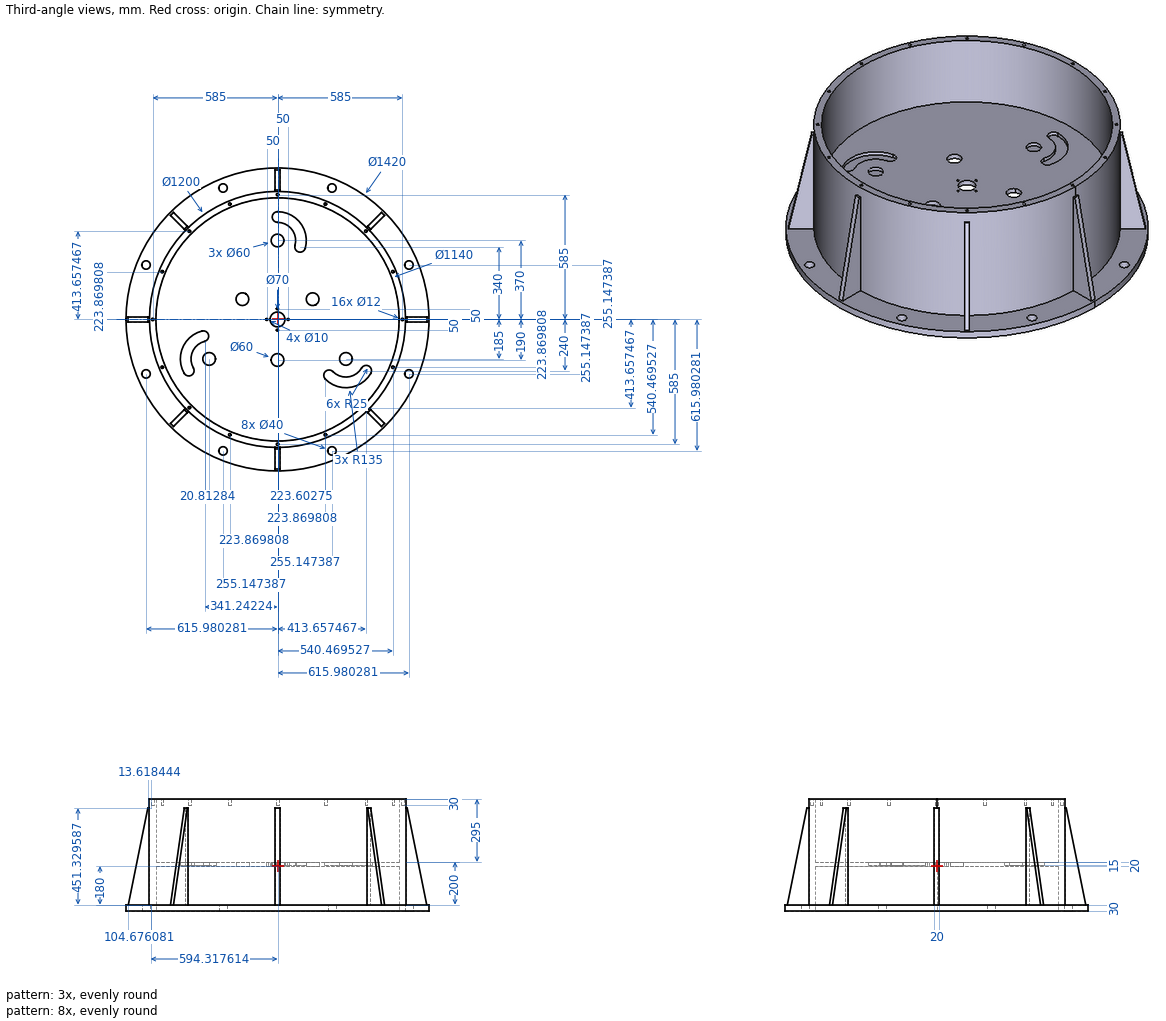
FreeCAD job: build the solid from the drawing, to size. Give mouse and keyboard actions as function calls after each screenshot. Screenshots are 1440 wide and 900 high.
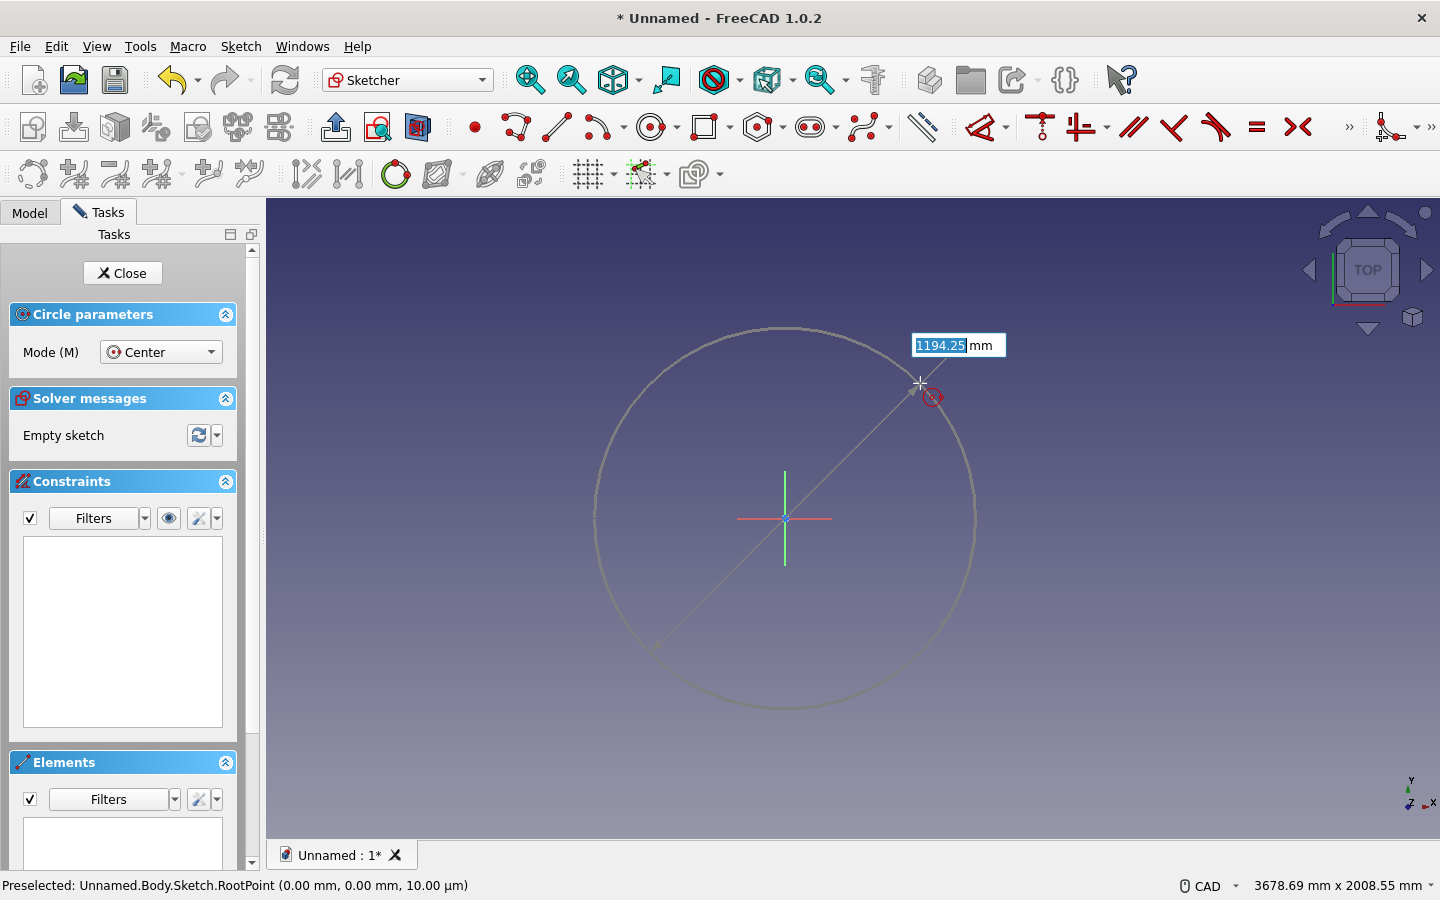
text(1200)
key(Return)
key(Escape)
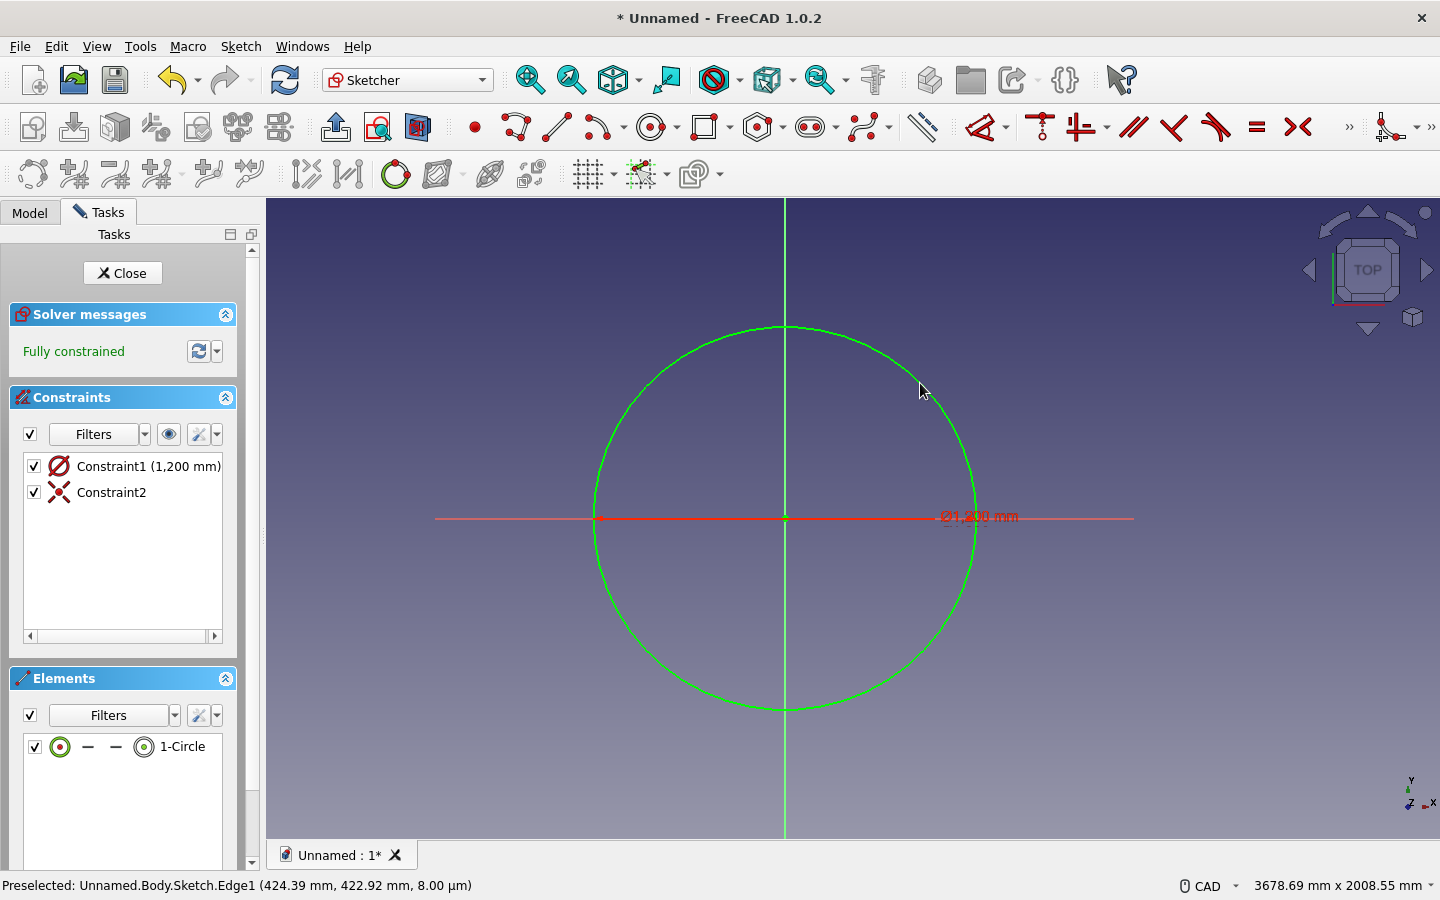
click(123, 273)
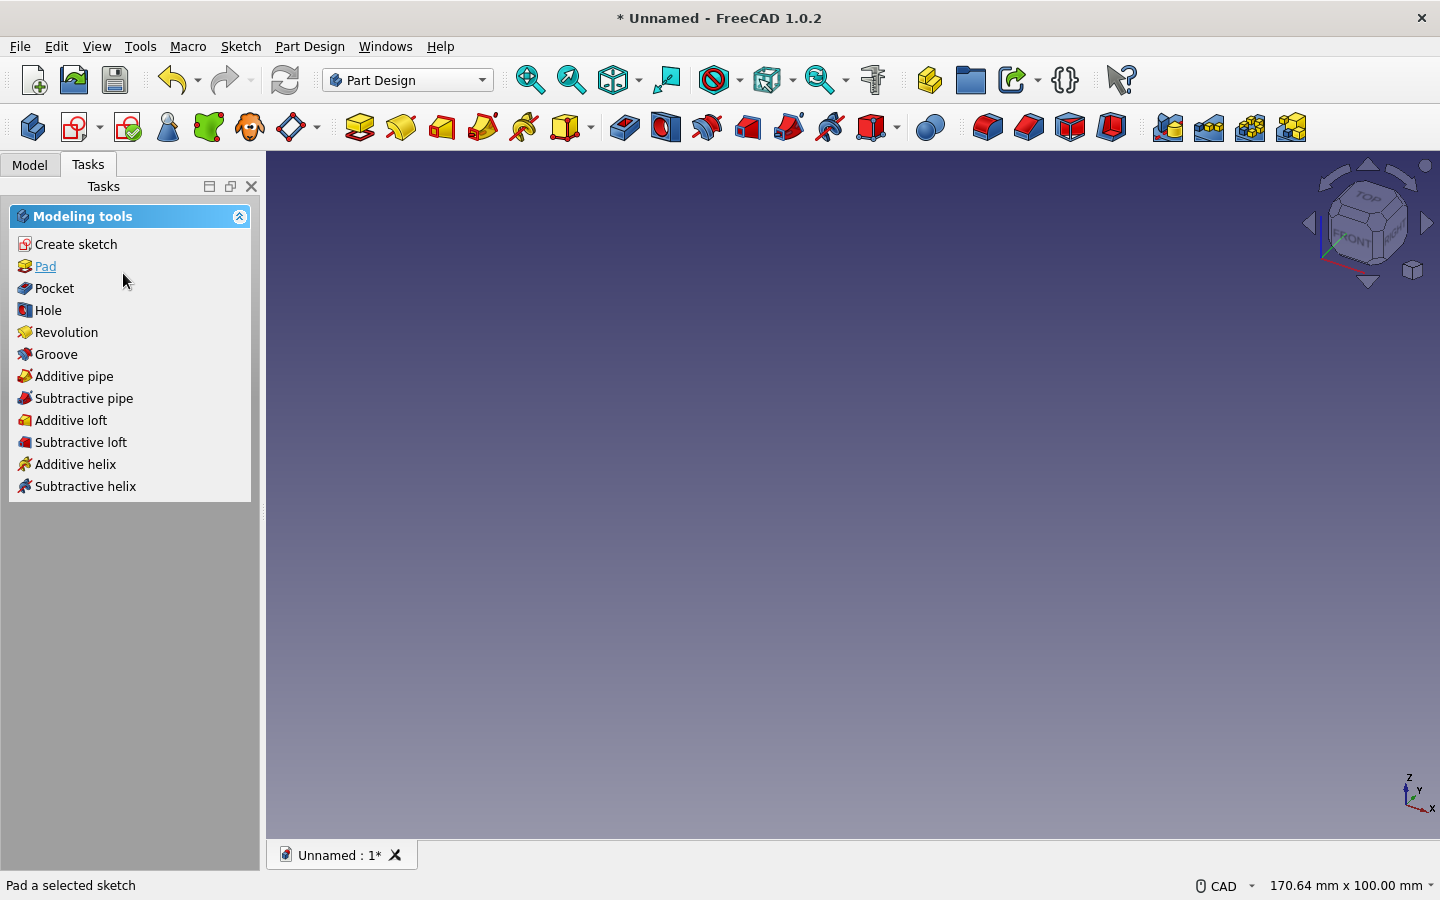
click(360, 128)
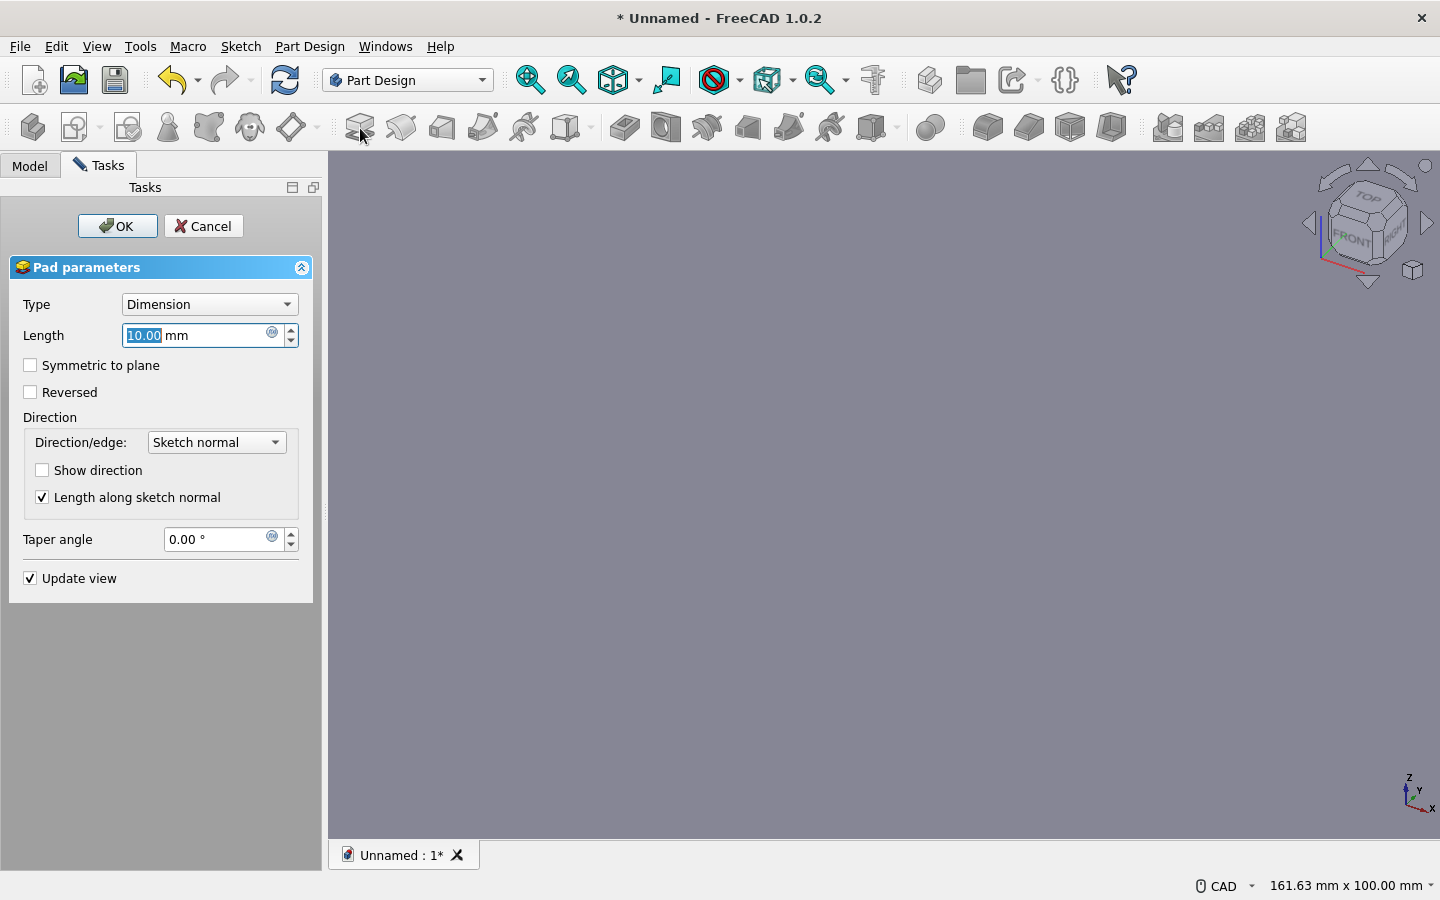
text(20)
key(Tab)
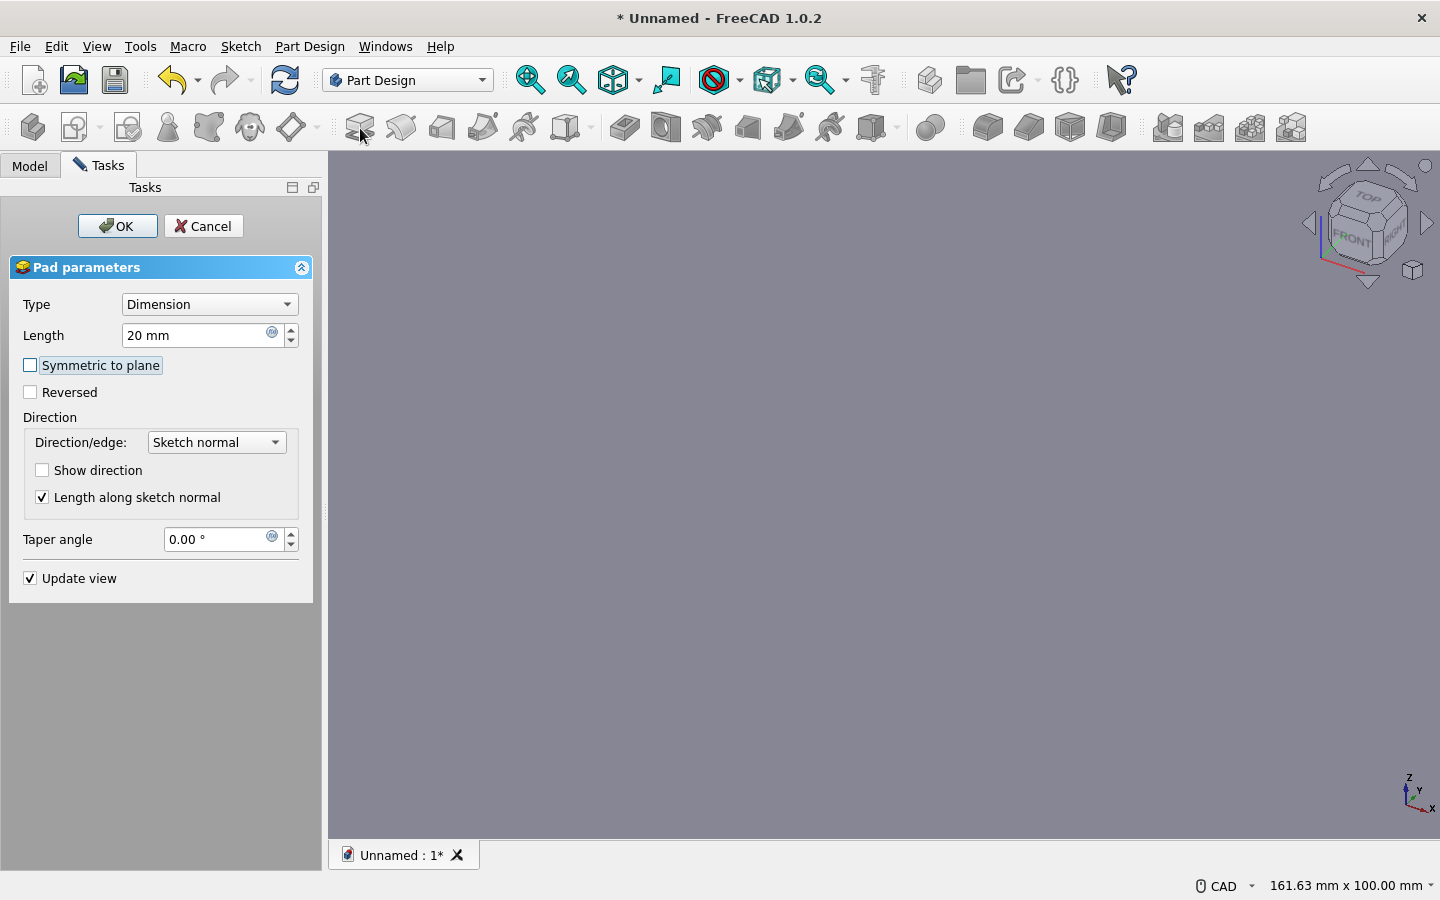
click(118, 226)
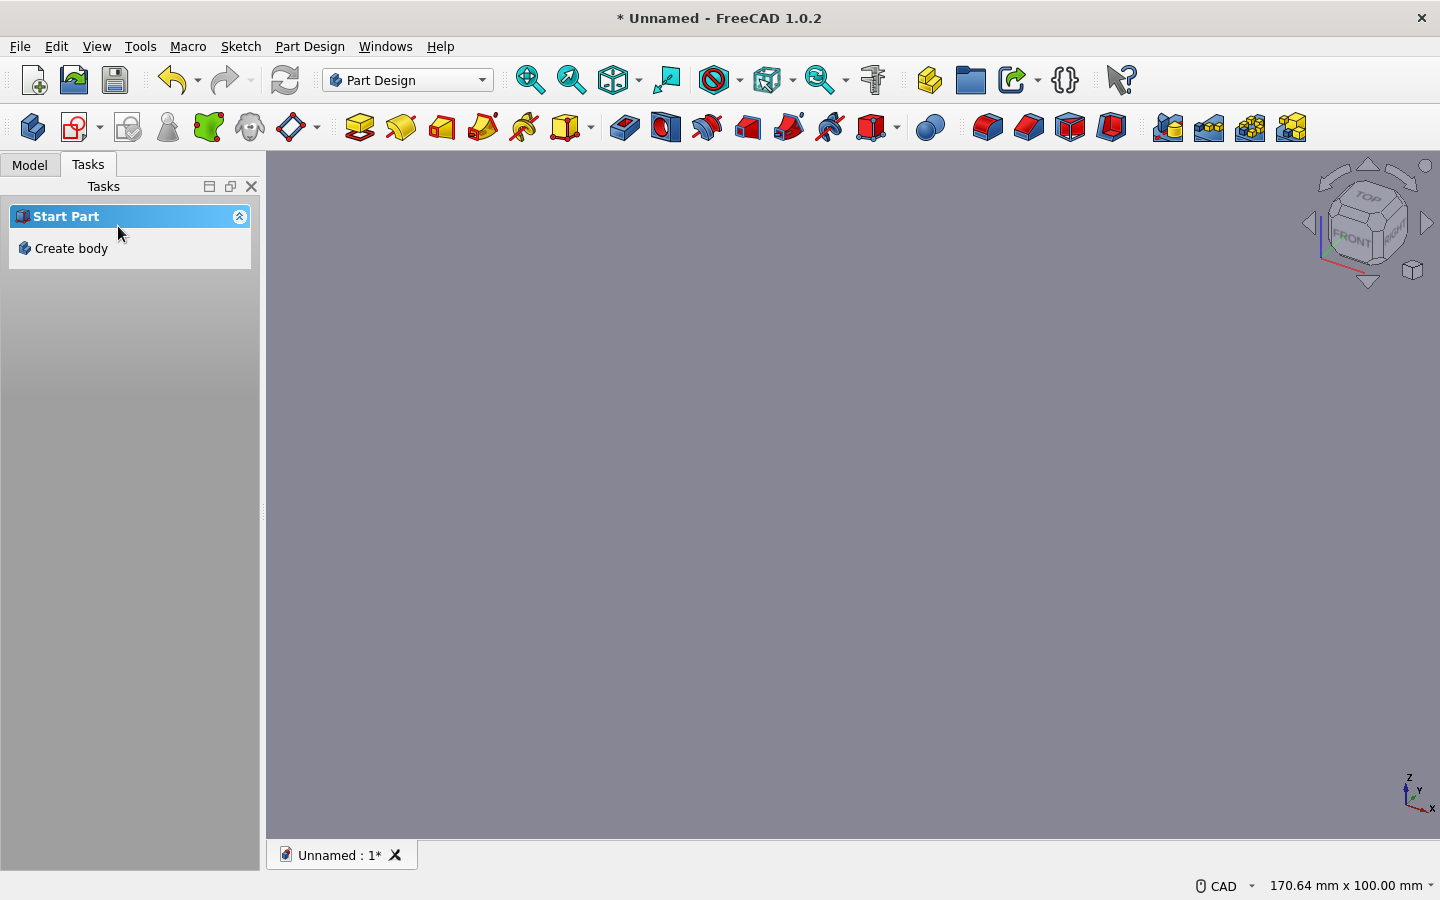
click(531, 80)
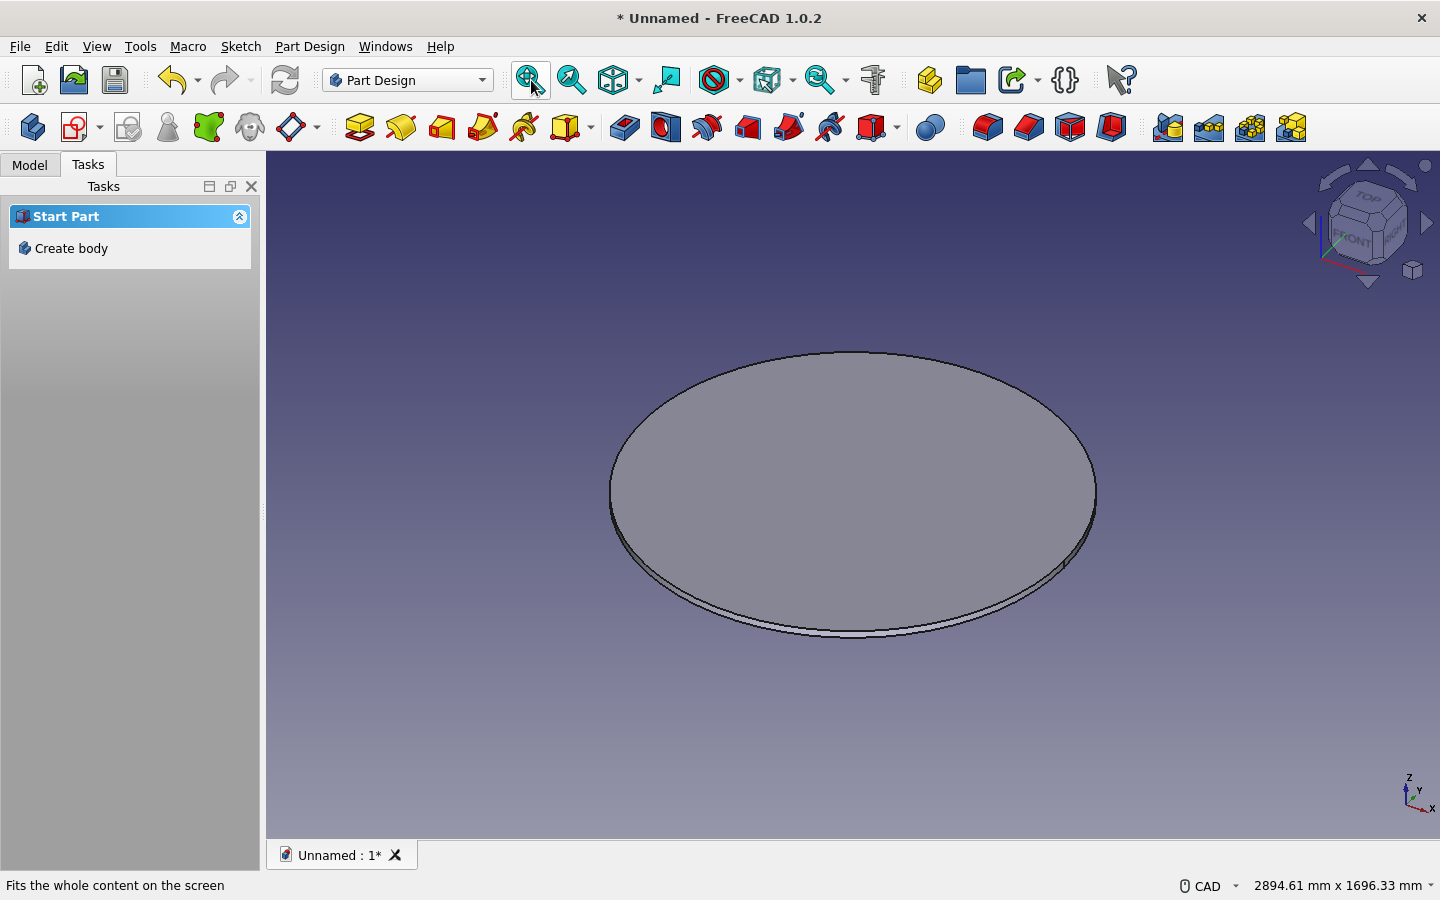
click(74, 128)